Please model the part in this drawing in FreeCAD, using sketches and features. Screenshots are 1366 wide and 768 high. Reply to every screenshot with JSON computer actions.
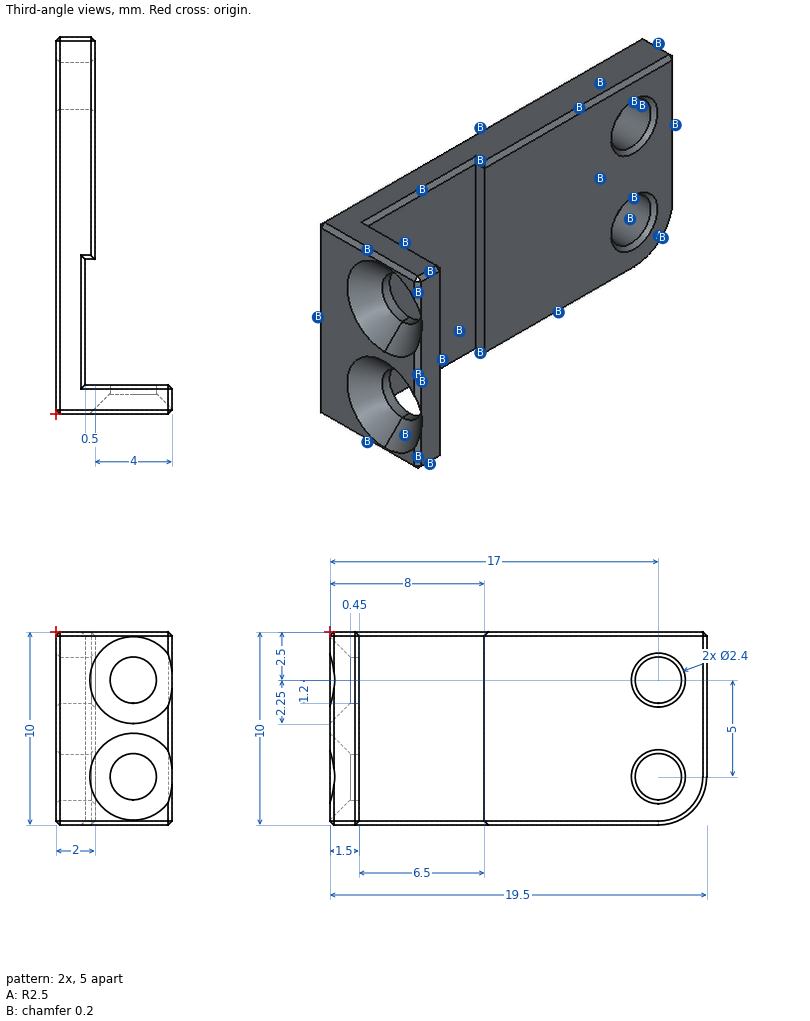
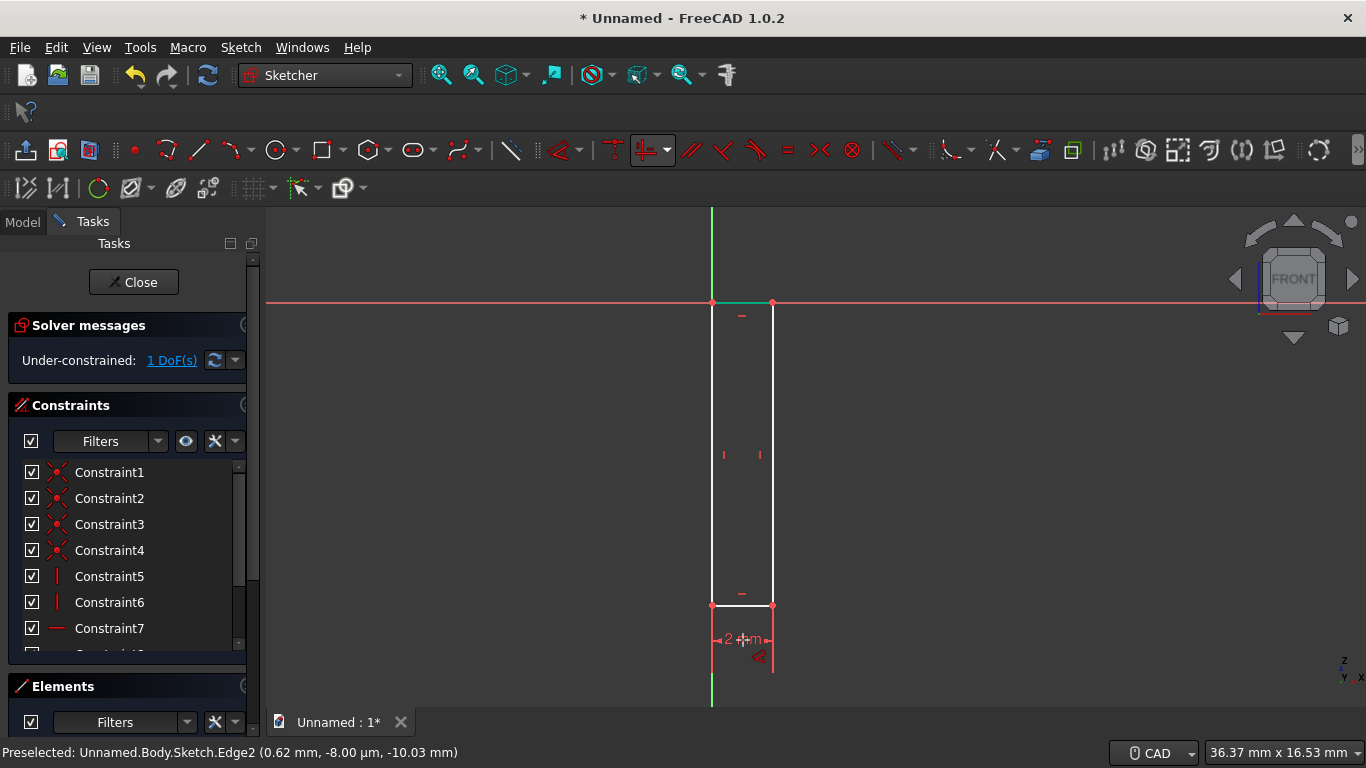
{"action": "left_click", "coordinate": [712, 394]}
{"action": "left_click", "coordinate": [678, 454]}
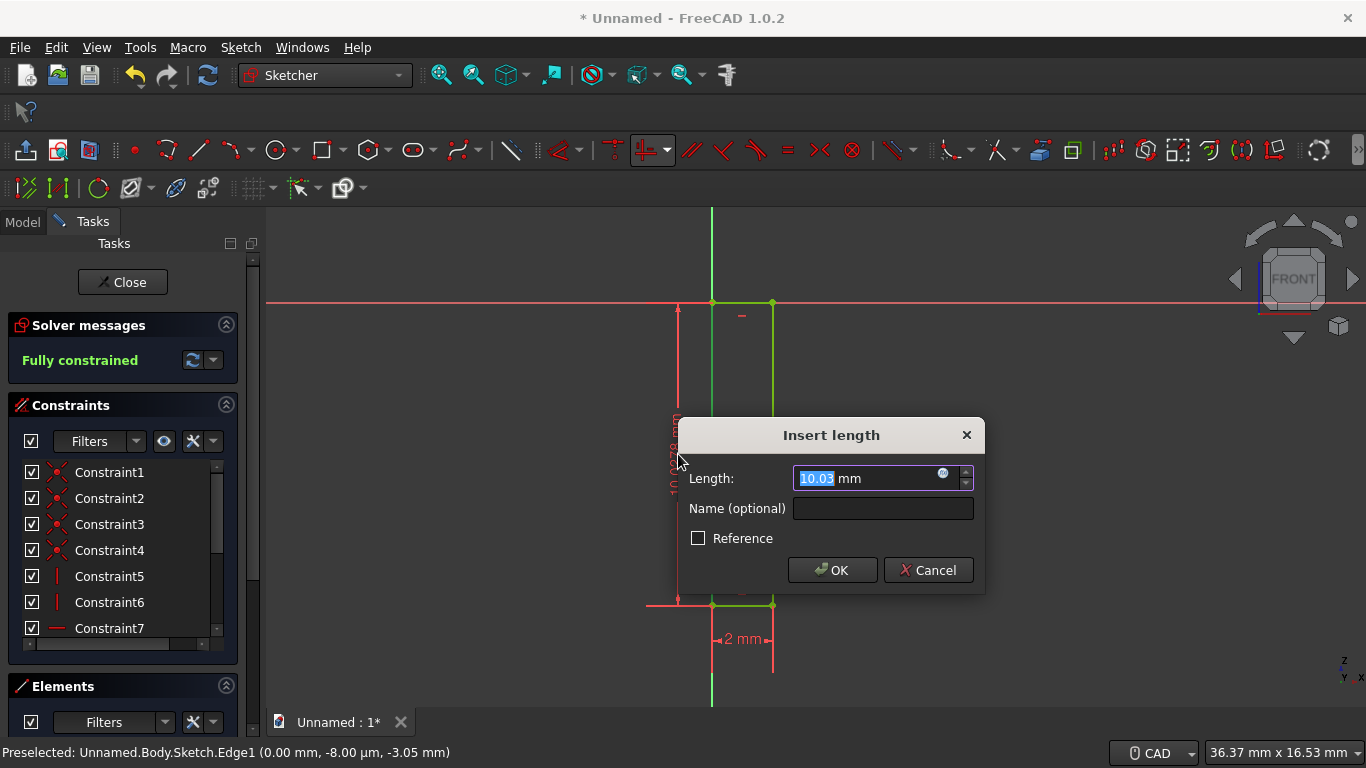
{"action": "type", "text": "10"}
{"action": "key", "text": "Return"}
{"action": "key", "text": "Escape"}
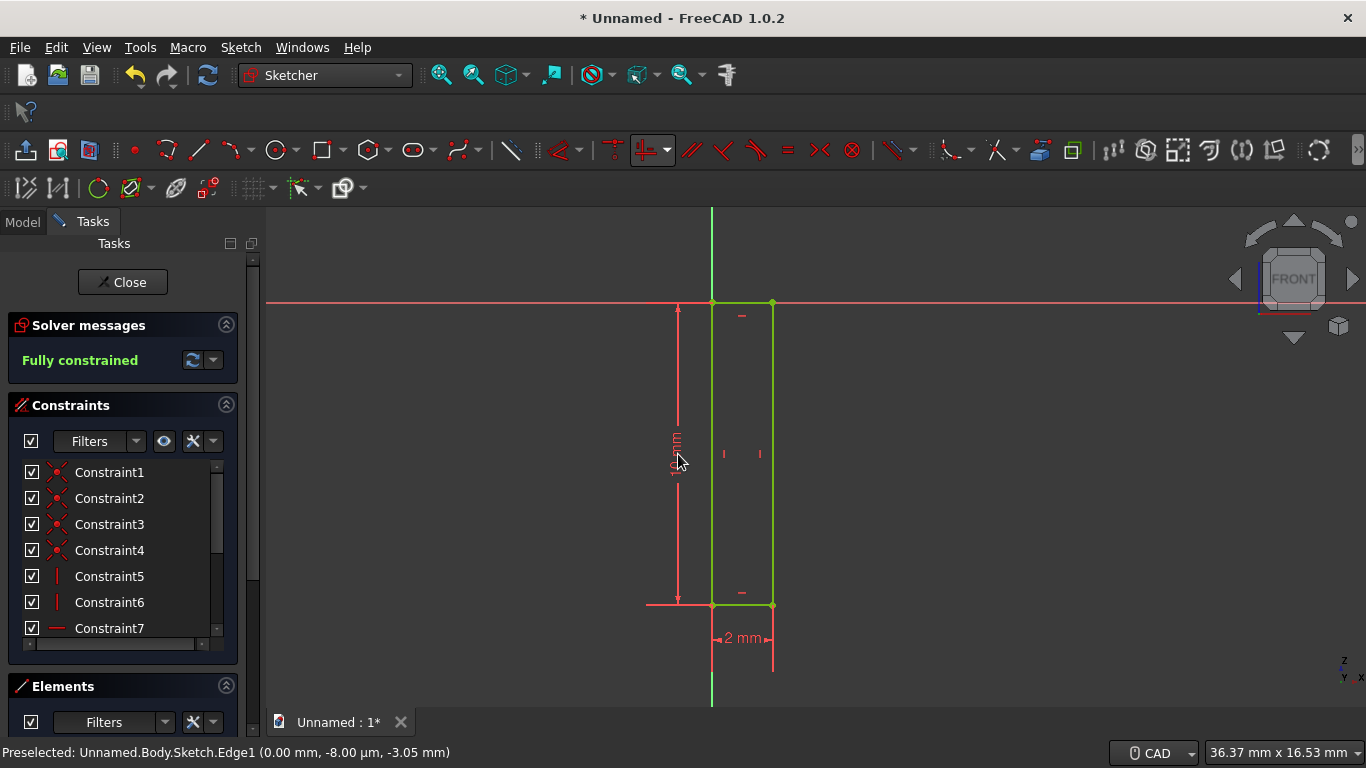
{"action": "left_click", "coordinate": [123, 282]}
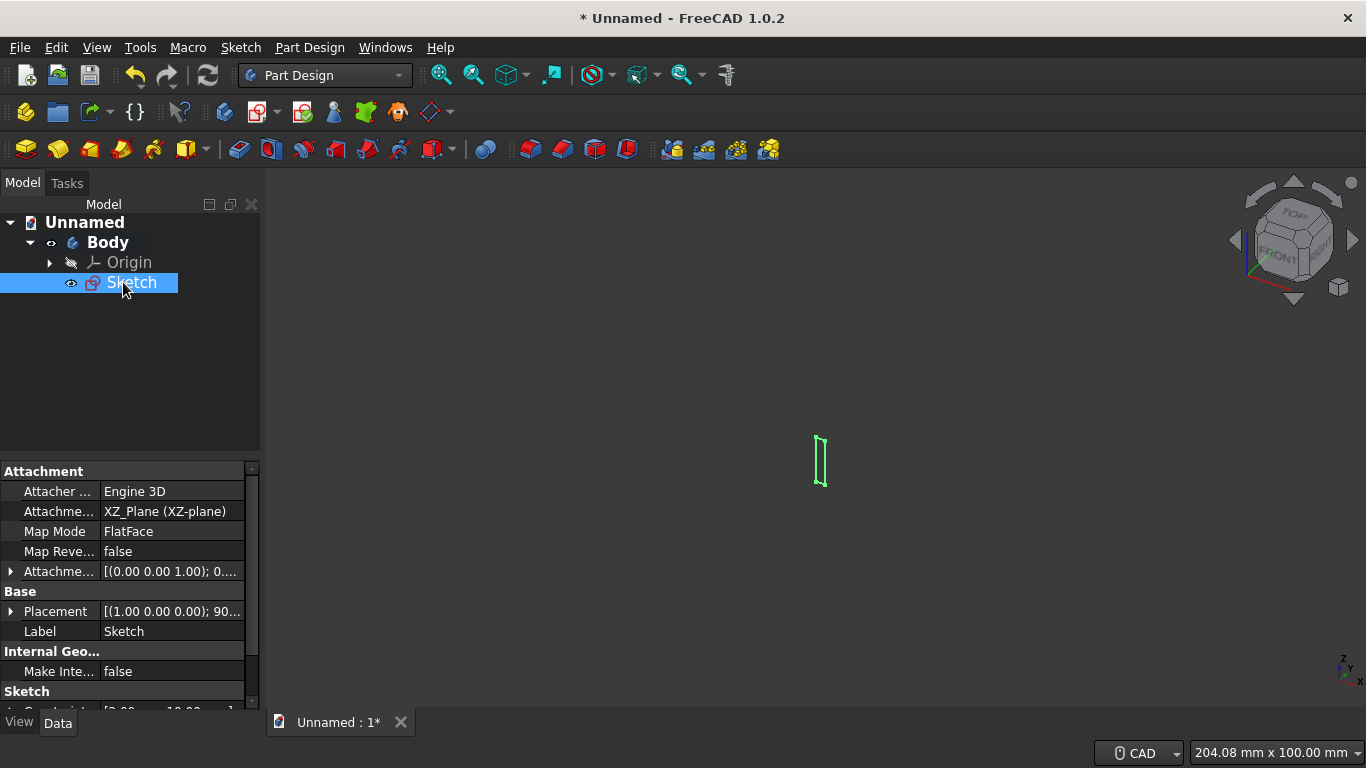
{"action": "left_click", "coordinate": [26, 150]}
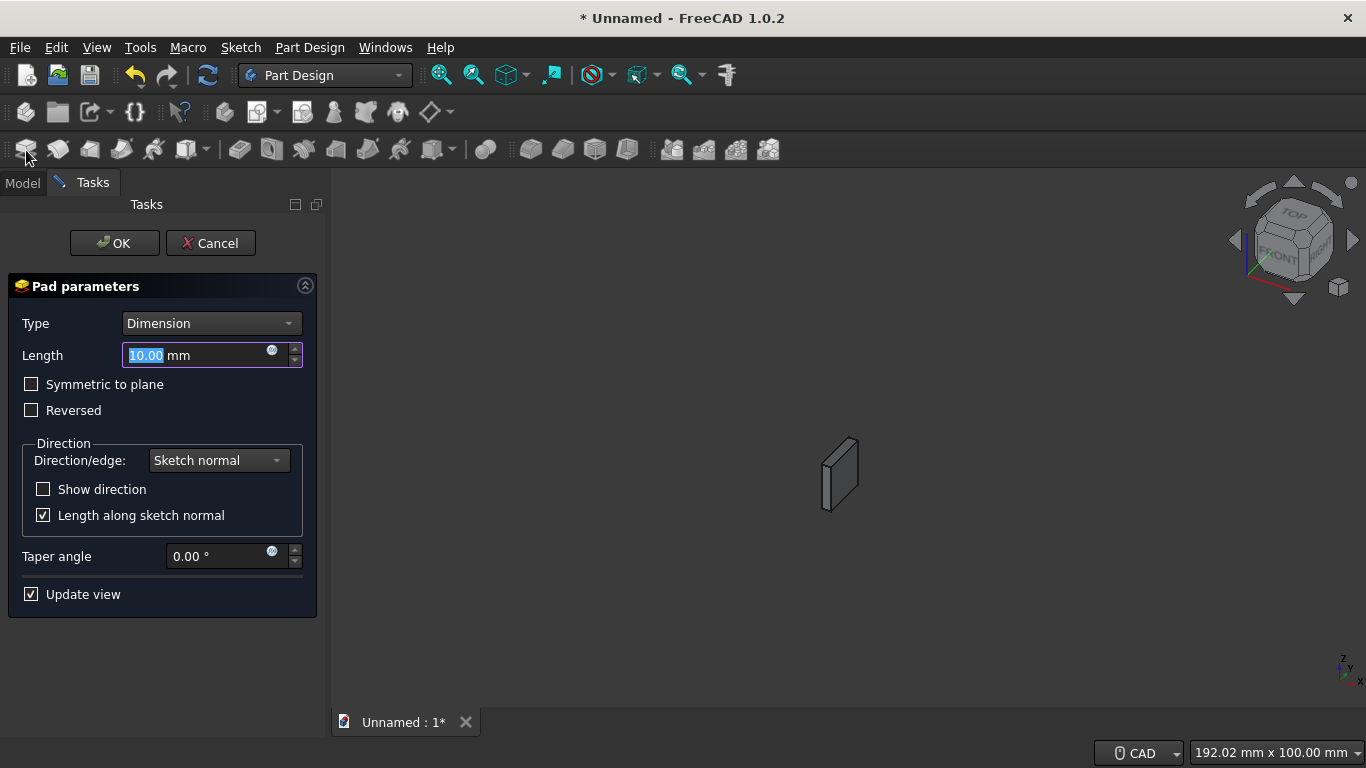
{"action": "type", "text": "19.5"}
{"action": "key", "text": "Tab"}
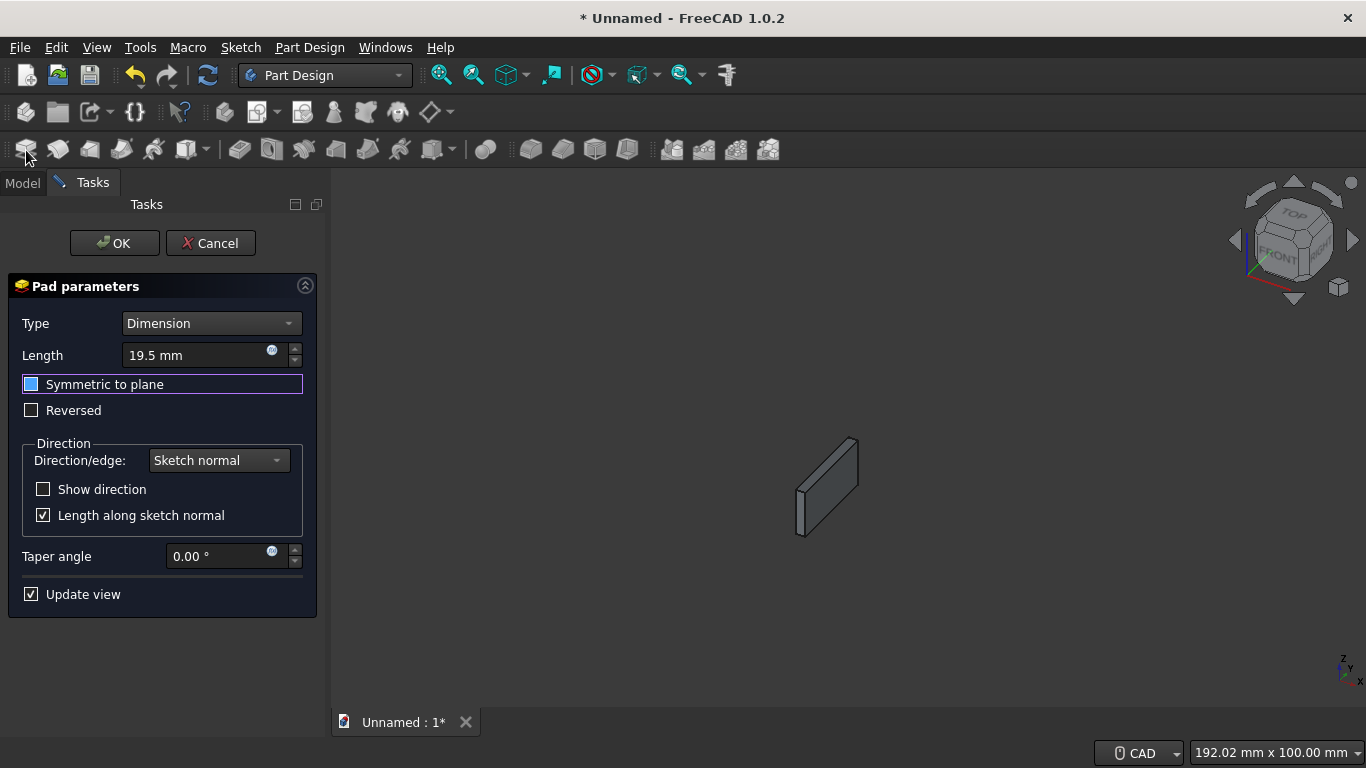
{"action": "left_click", "coordinate": [30, 410]}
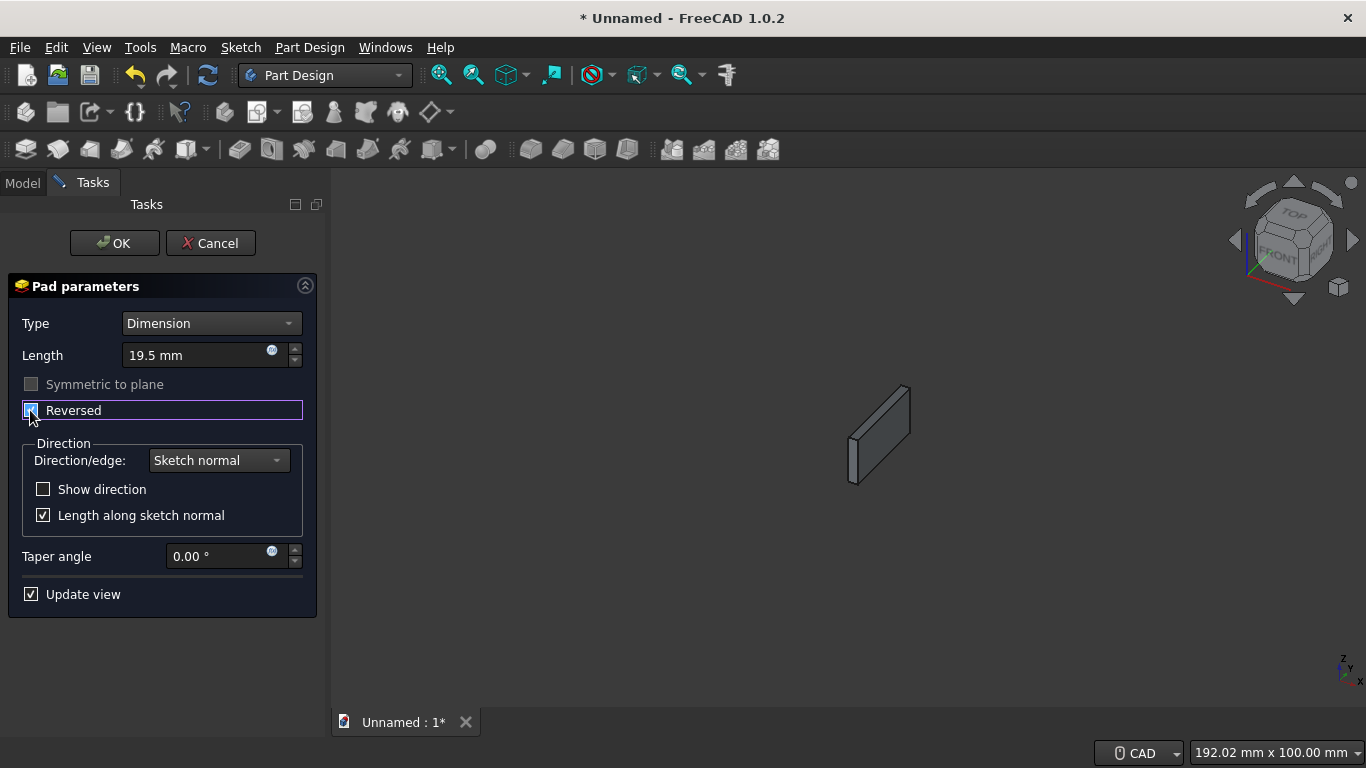
{"action": "left_click", "coordinate": [115, 243]}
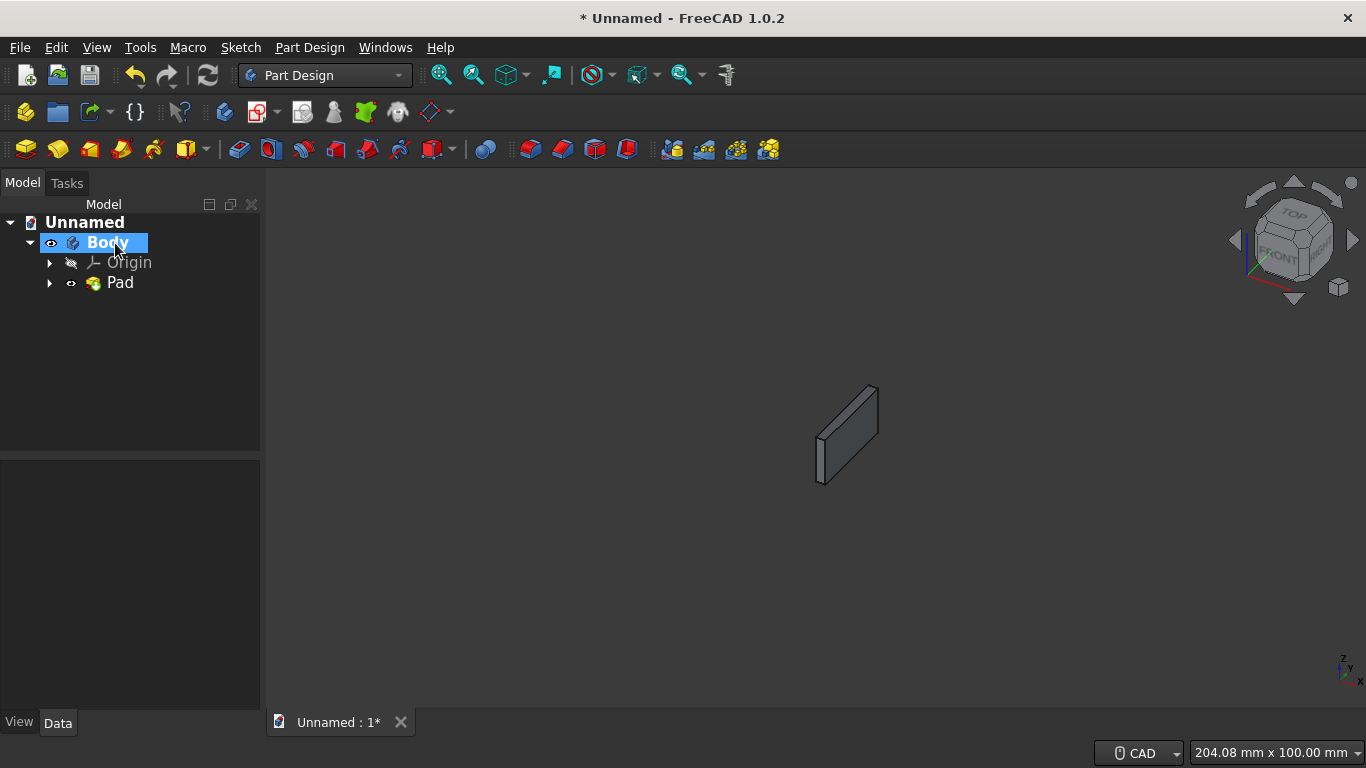
{"action": "left_click", "coordinate": [442, 76]}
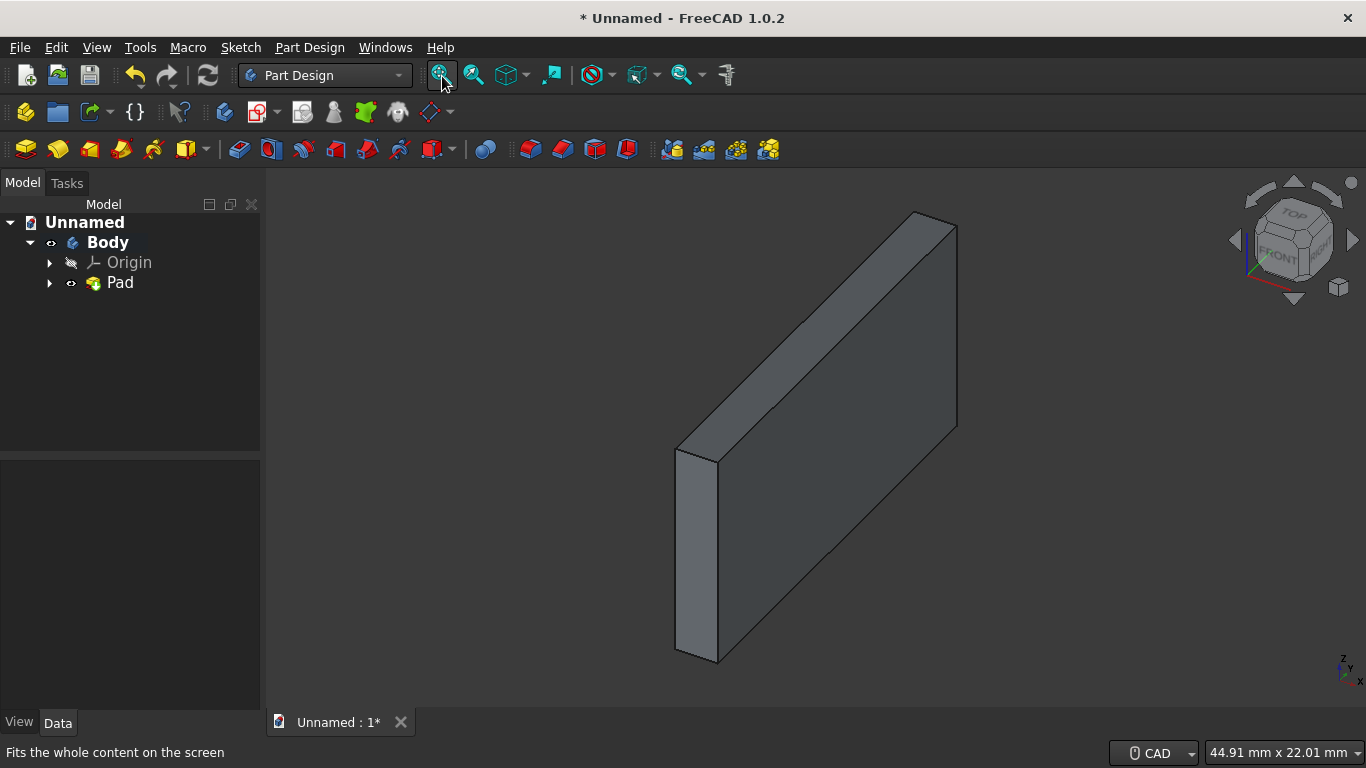
{"action": "left_click", "coordinate": [871, 410]}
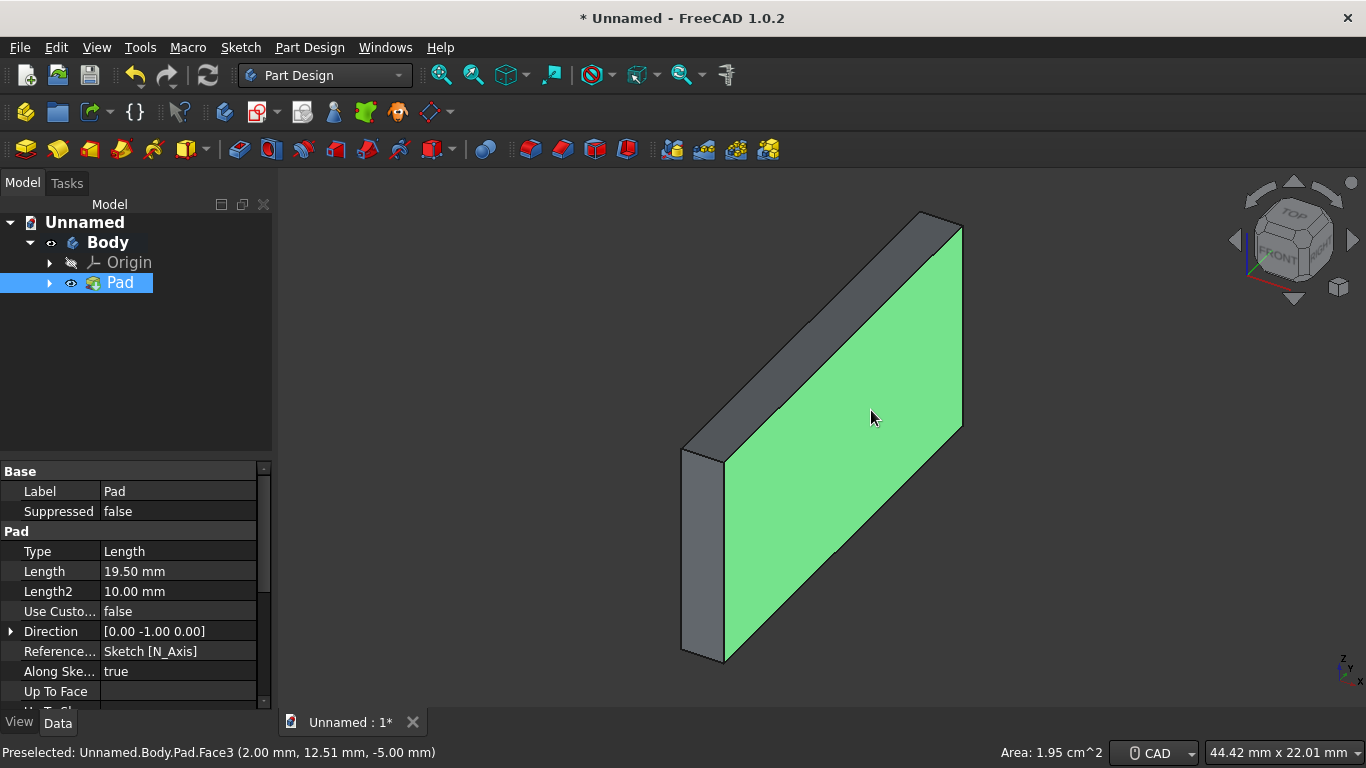
{"action": "left_click", "coordinate": [258, 112]}